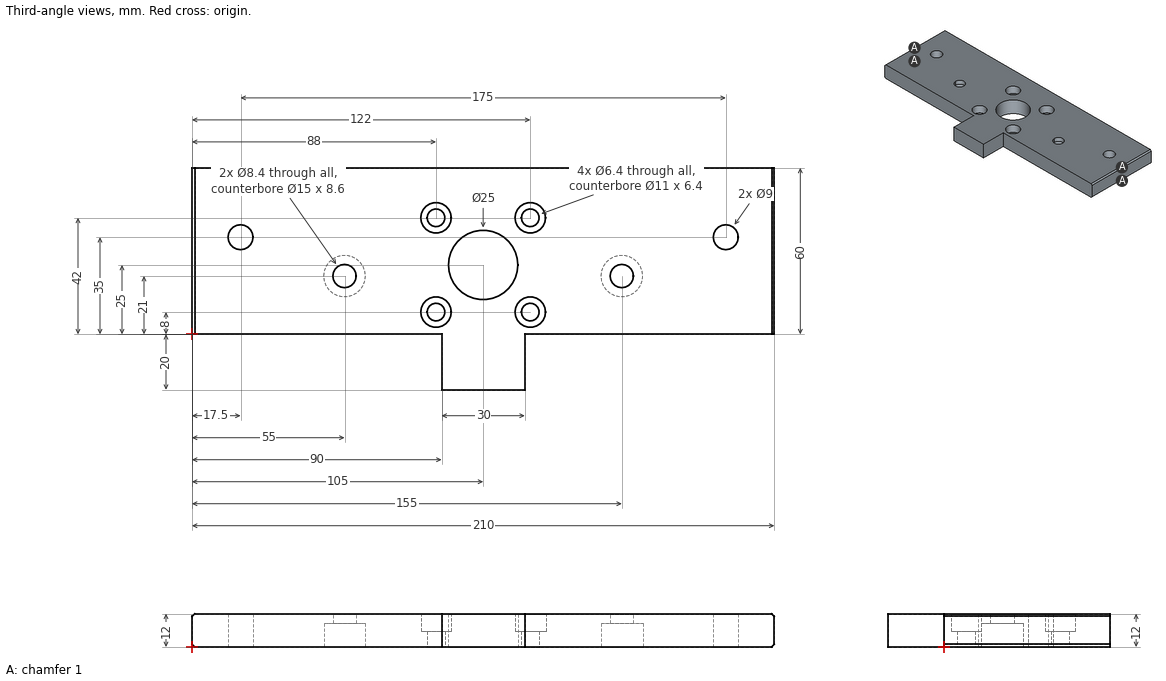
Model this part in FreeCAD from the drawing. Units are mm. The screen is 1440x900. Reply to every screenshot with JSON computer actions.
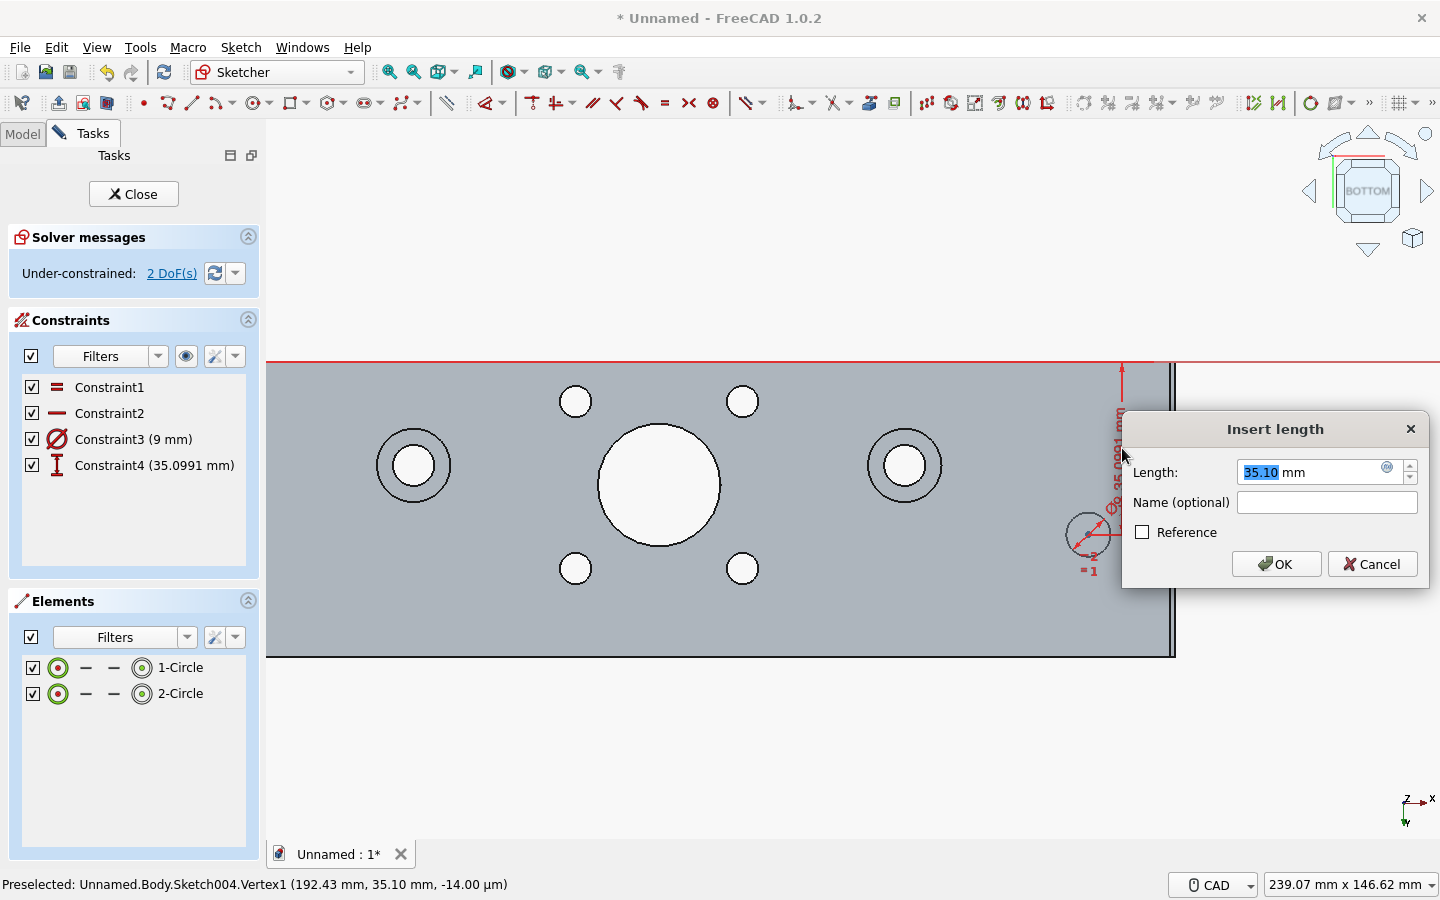
{"action": "type", "text": "35"}
{"action": "key", "text": "Return"}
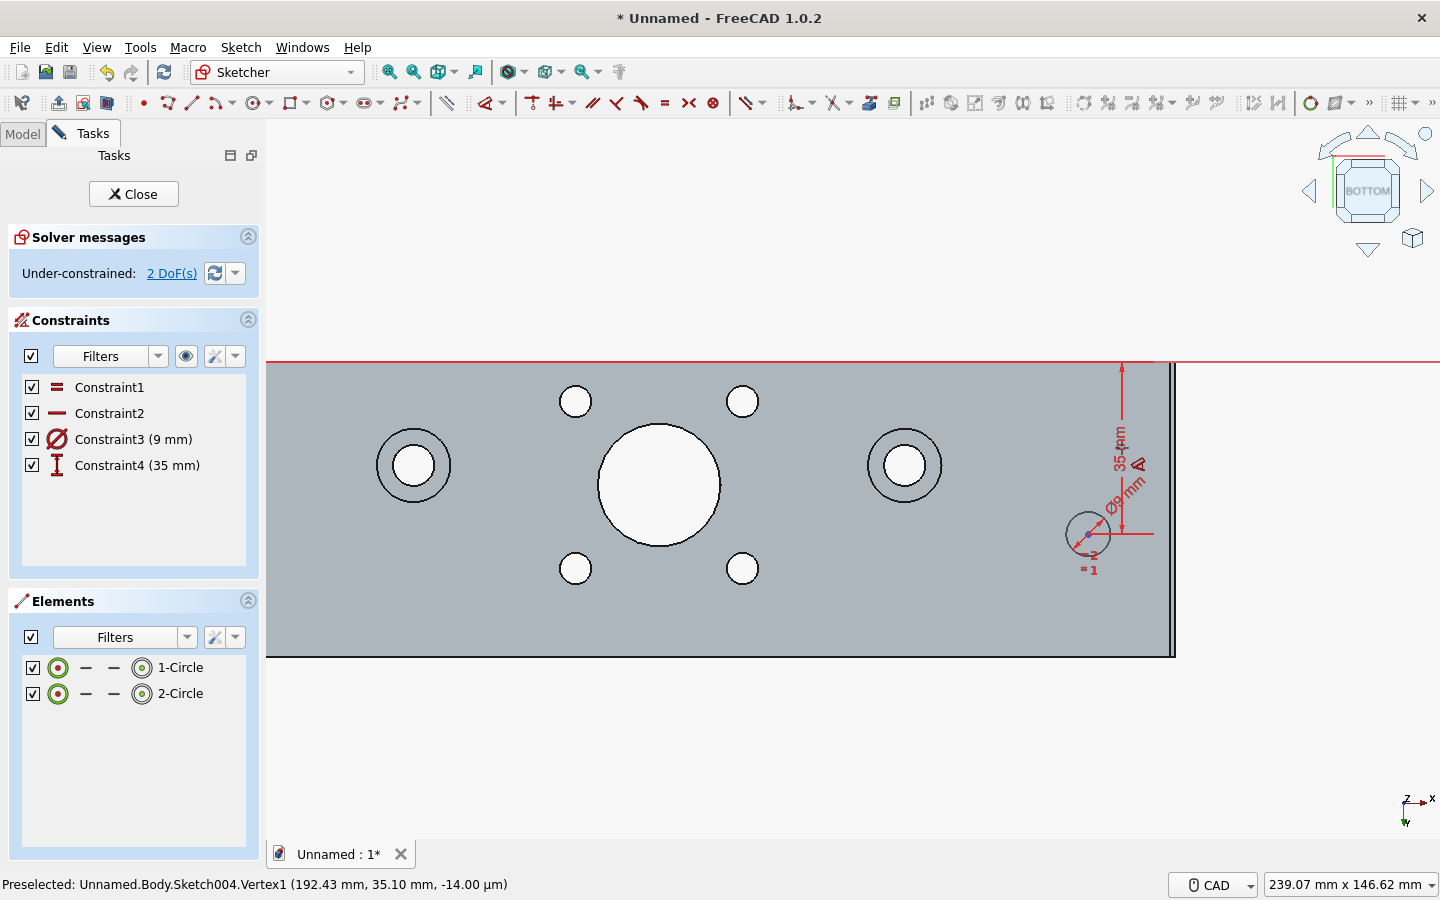
{"action": "scroll", "coordinate": [1104, 519], "scroll_direction": "down", "scroll_amount": 2}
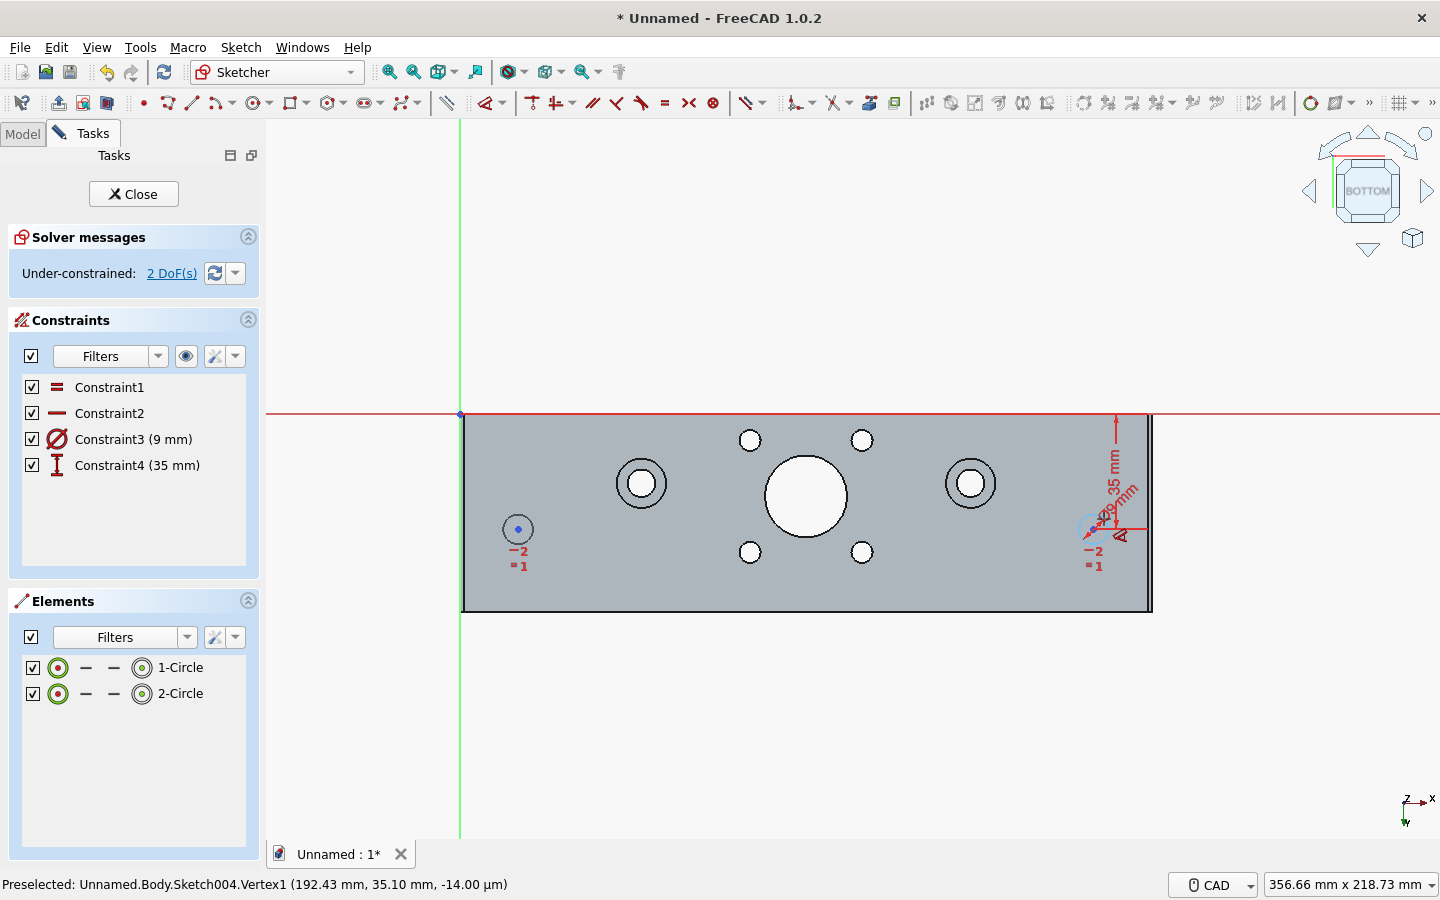
{"action": "left_click", "coordinate": [518, 529]}
{"action": "left_click", "coordinate": [489, 380]}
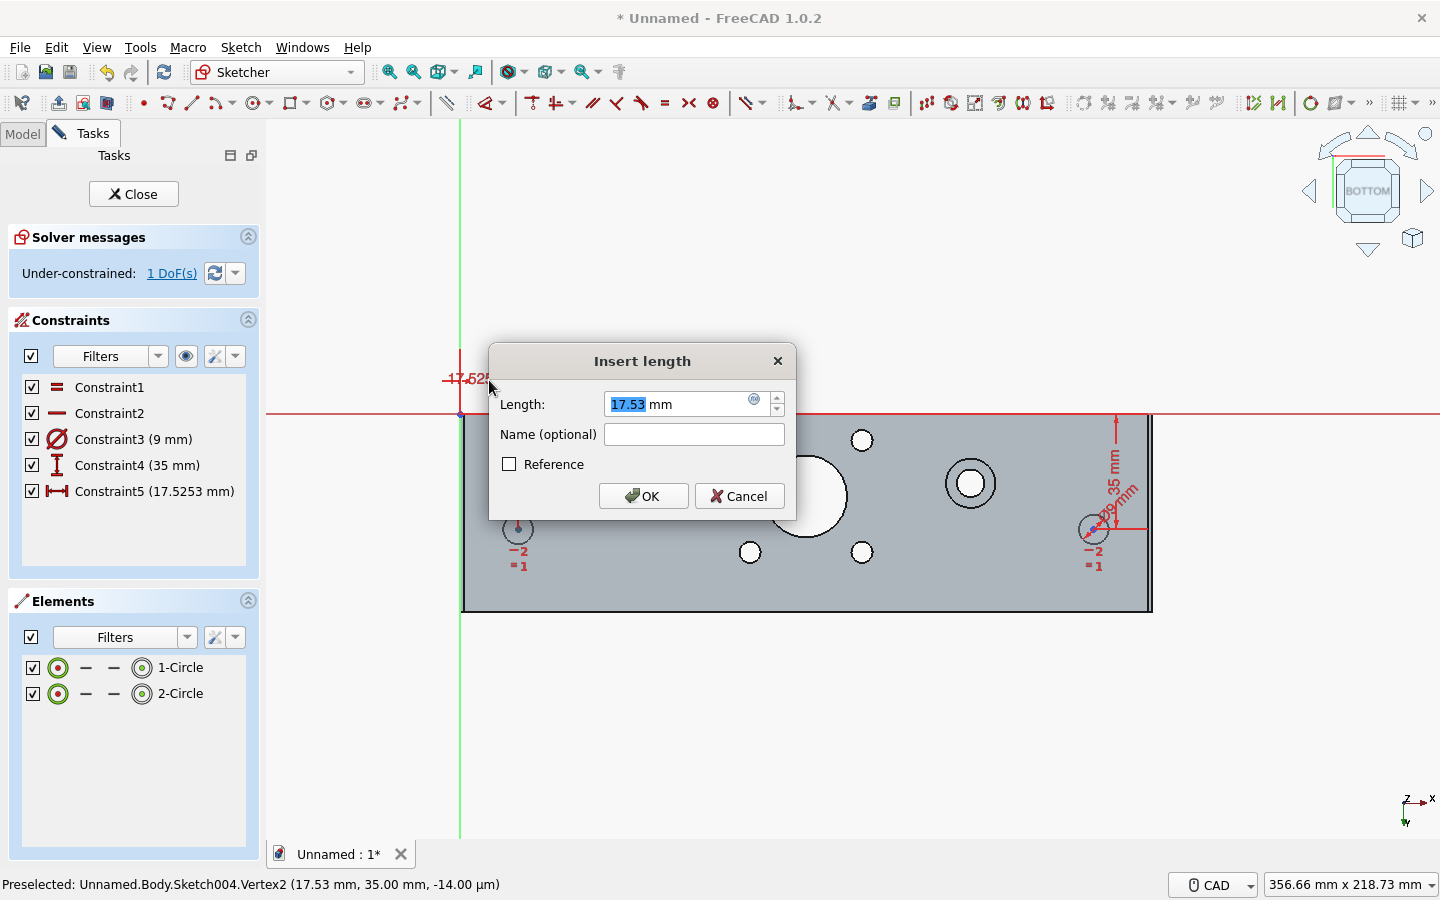
{"action": "type", "text": "17.5"}
{"action": "key", "text": "Return"}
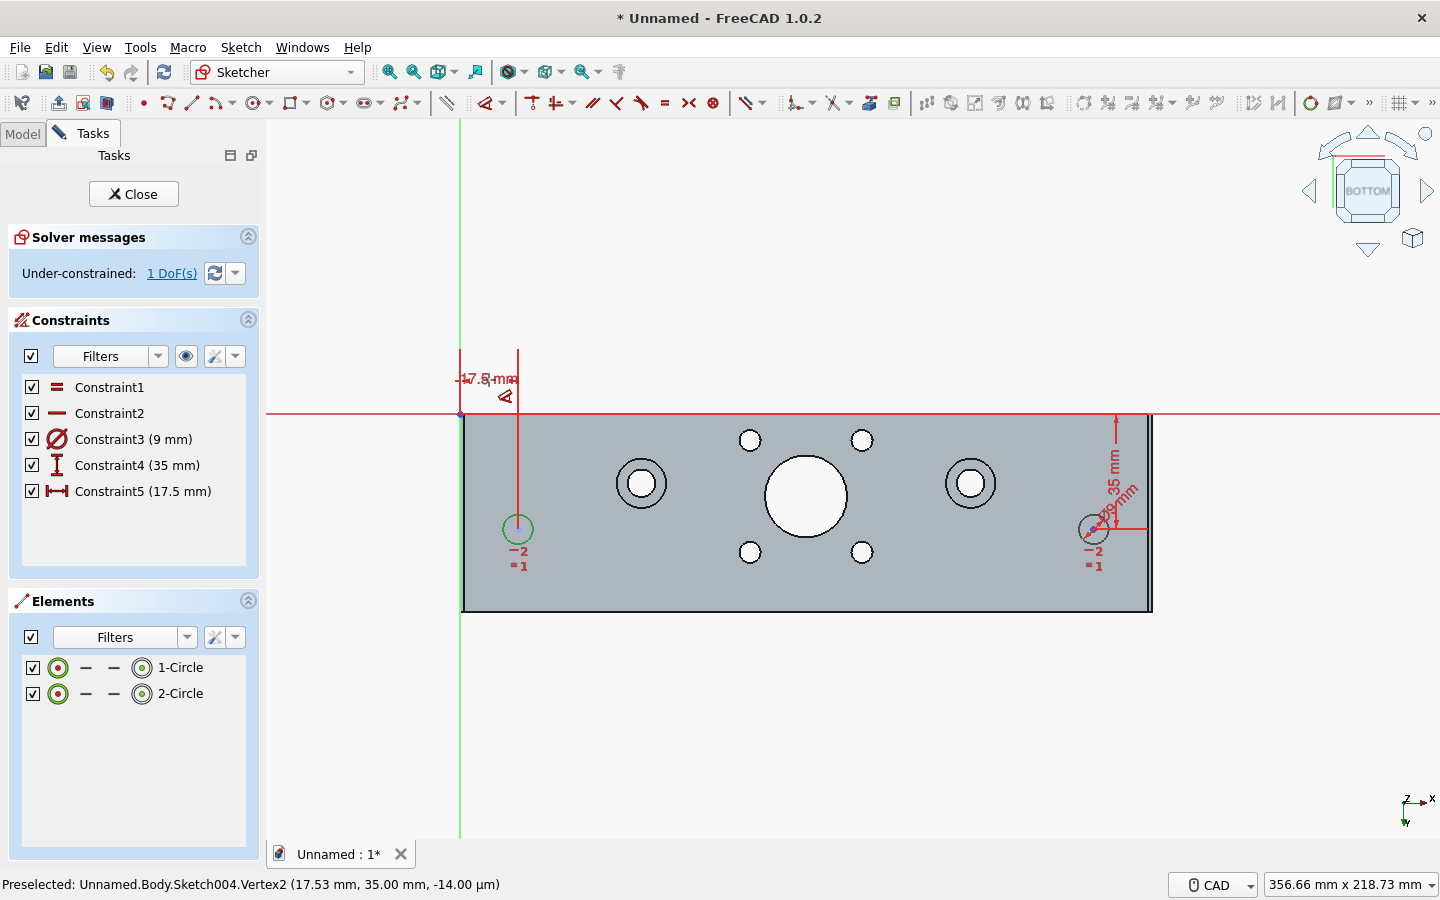
{"action": "left_click", "coordinate": [1094, 529]}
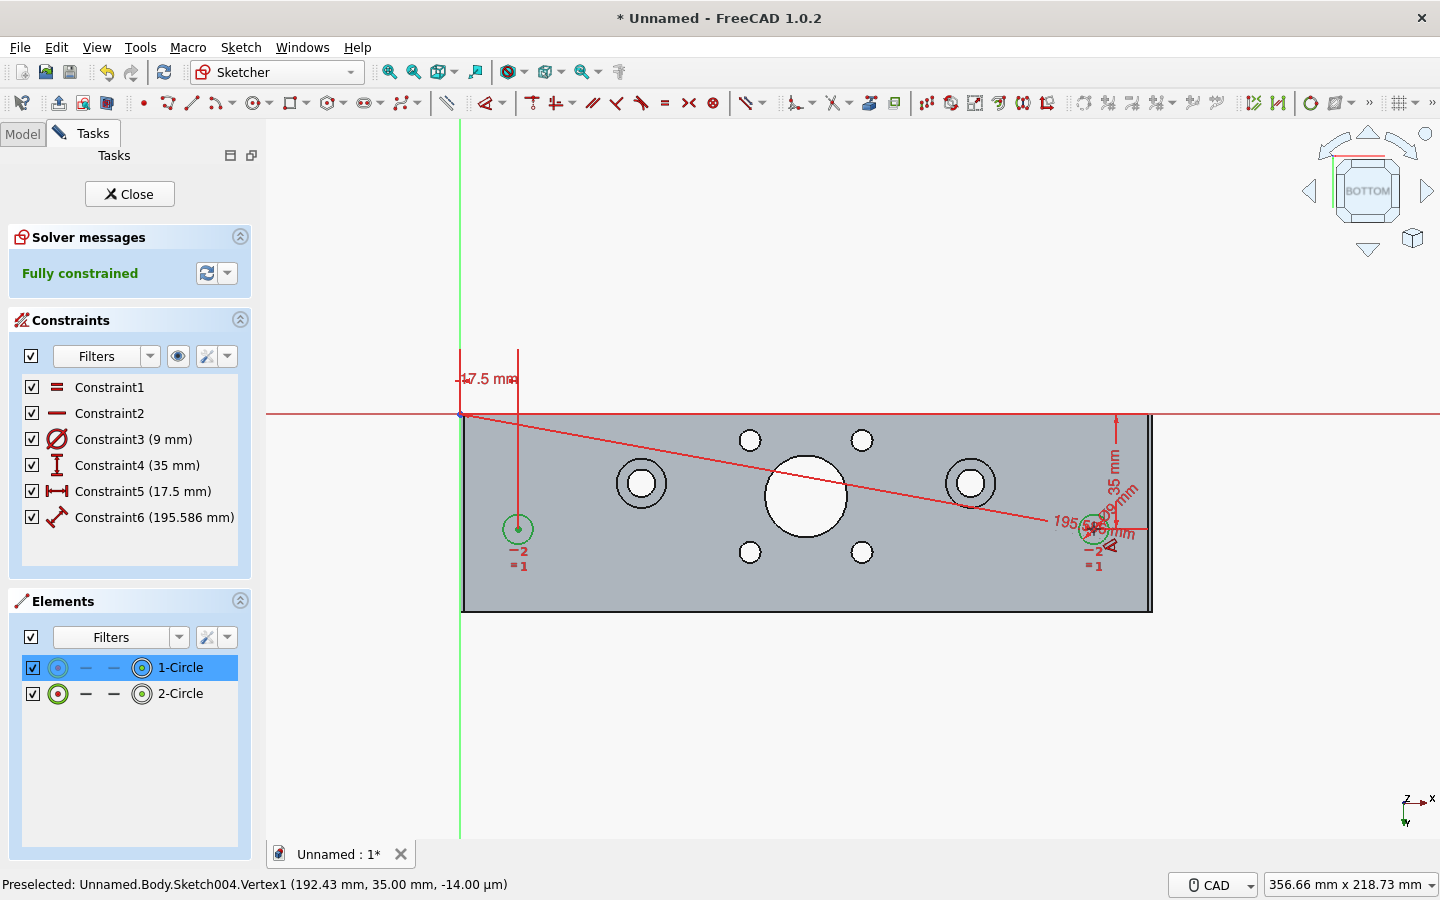
{"action": "left_click", "coordinate": [518, 529]}
{"action": "left_click", "coordinate": [806, 563]}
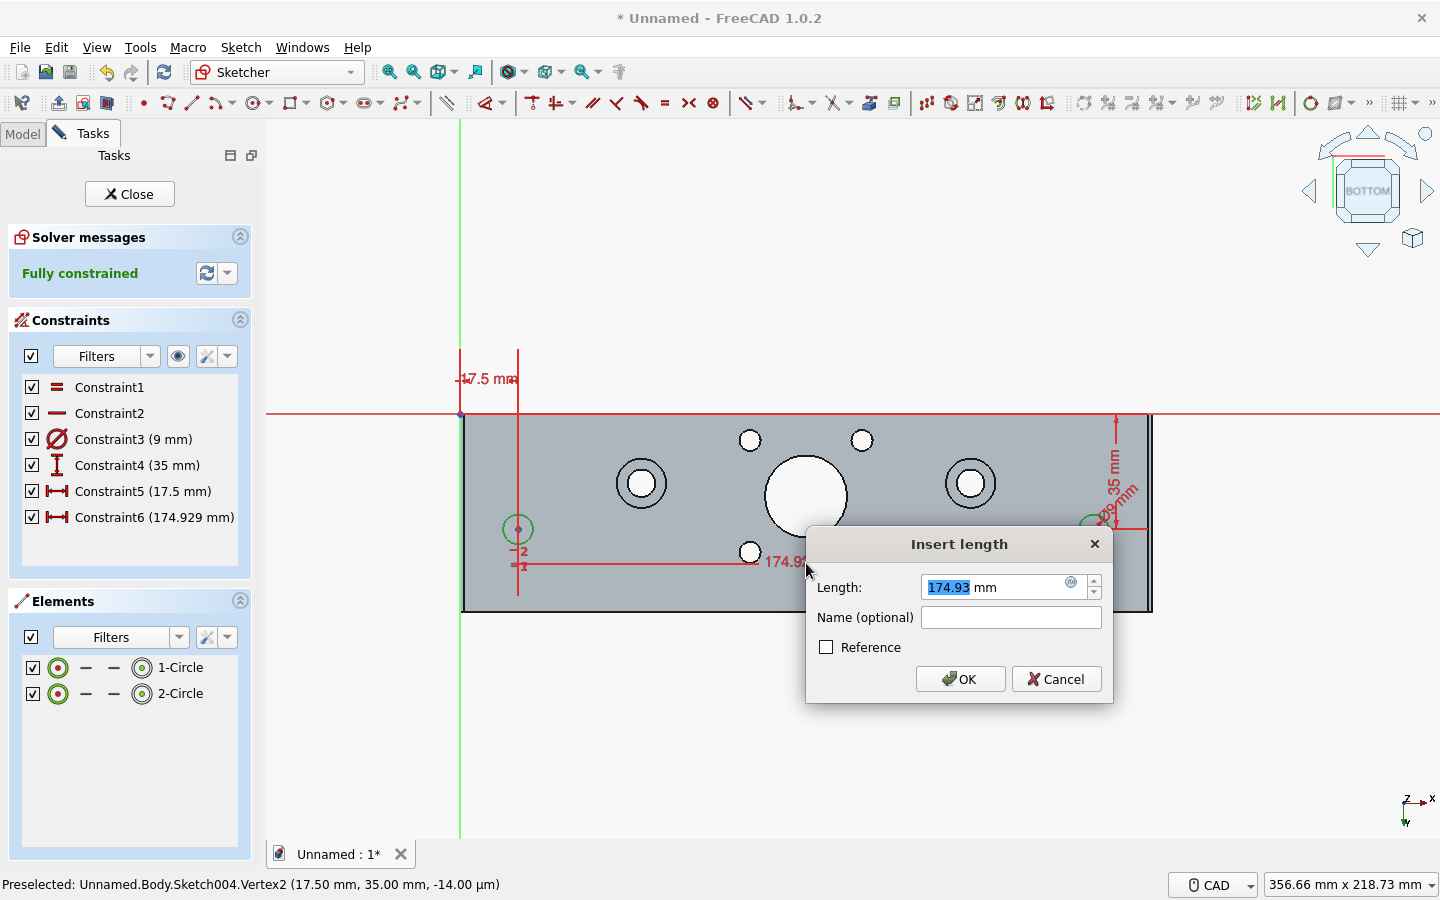
{"action": "type", "text": "175"}
{"action": "key", "text": "Return"}
{"action": "key", "text": "Escape"}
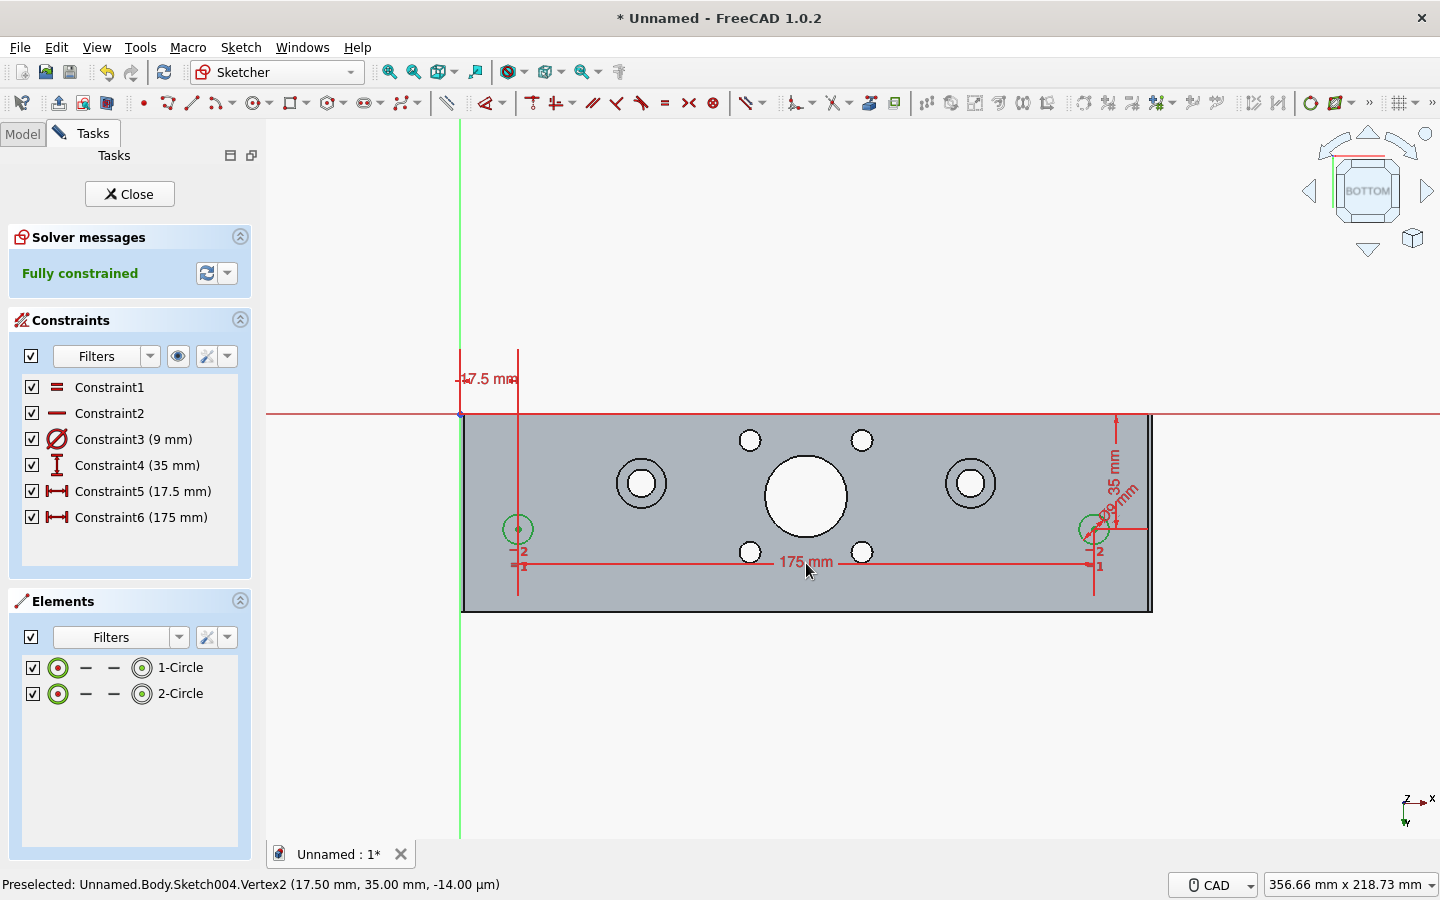
{"action": "left_click", "coordinate": [130, 194]}